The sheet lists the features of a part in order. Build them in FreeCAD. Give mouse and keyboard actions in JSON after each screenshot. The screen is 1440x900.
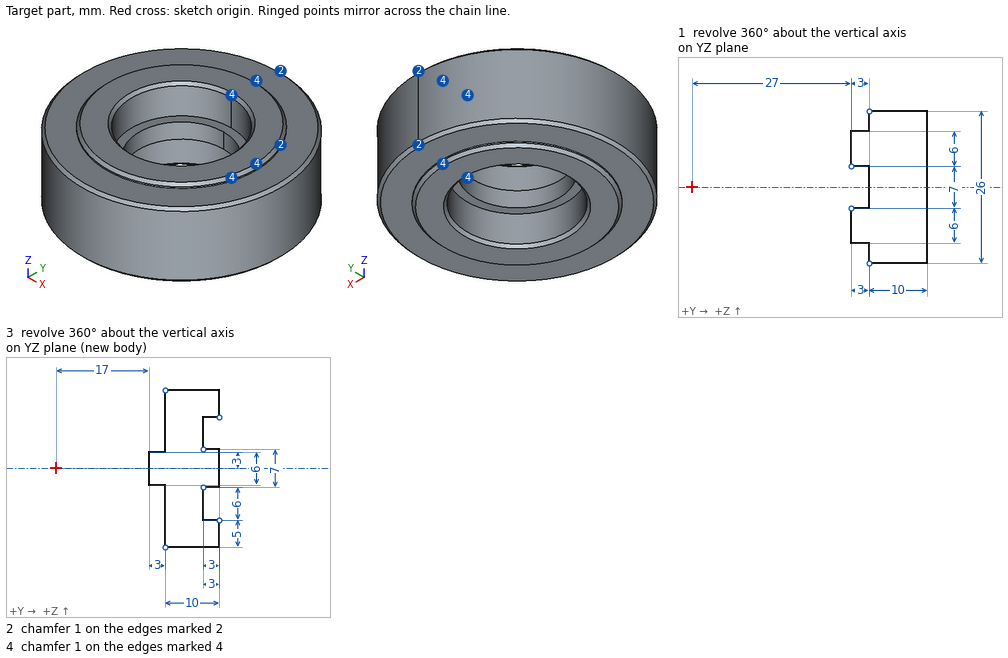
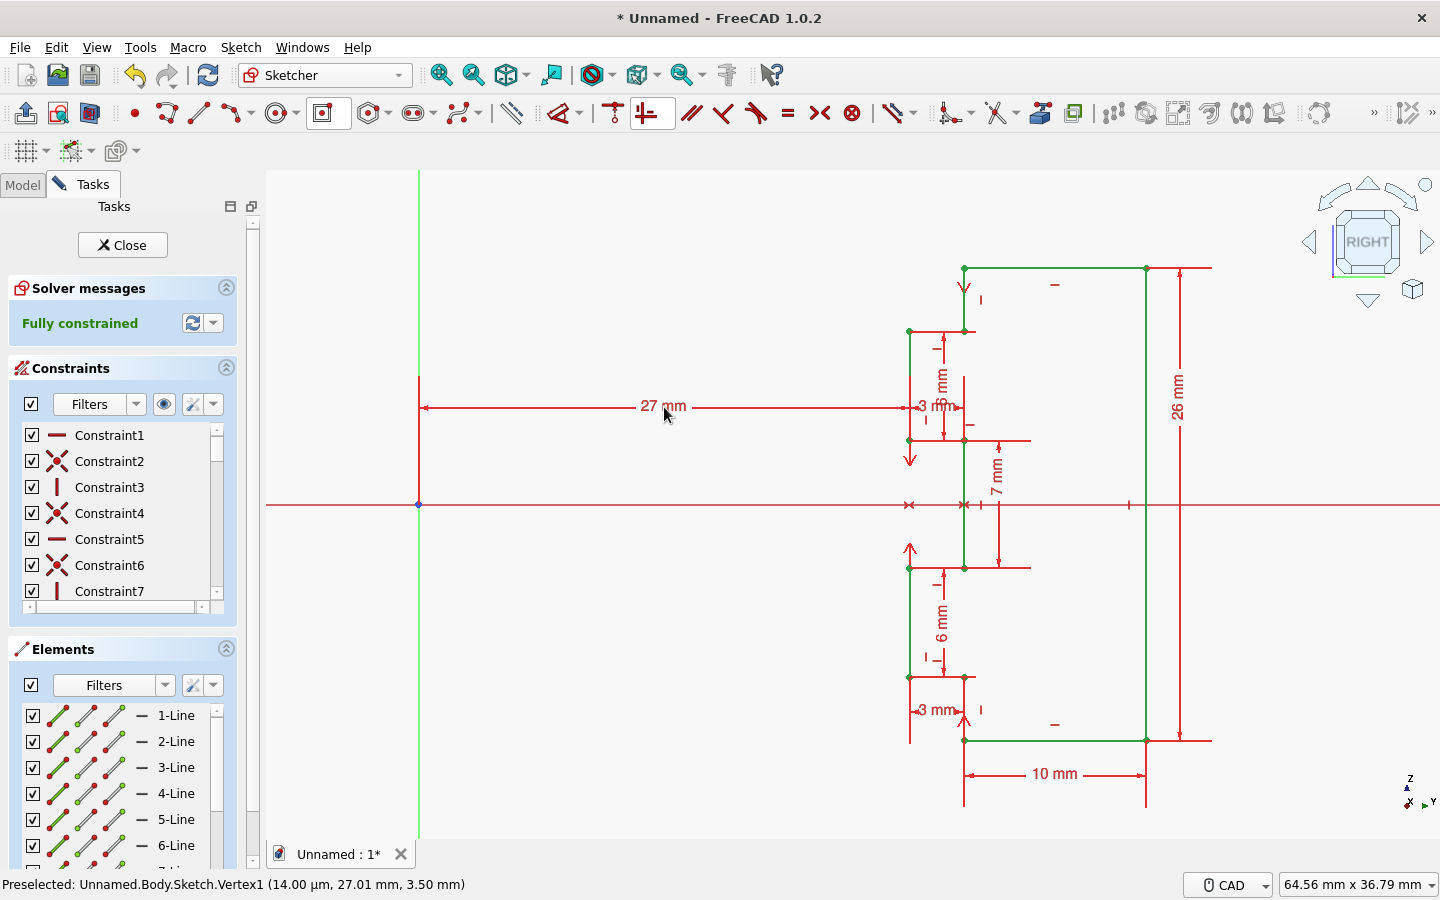
{"action": "left_click", "coordinate": [123, 245]}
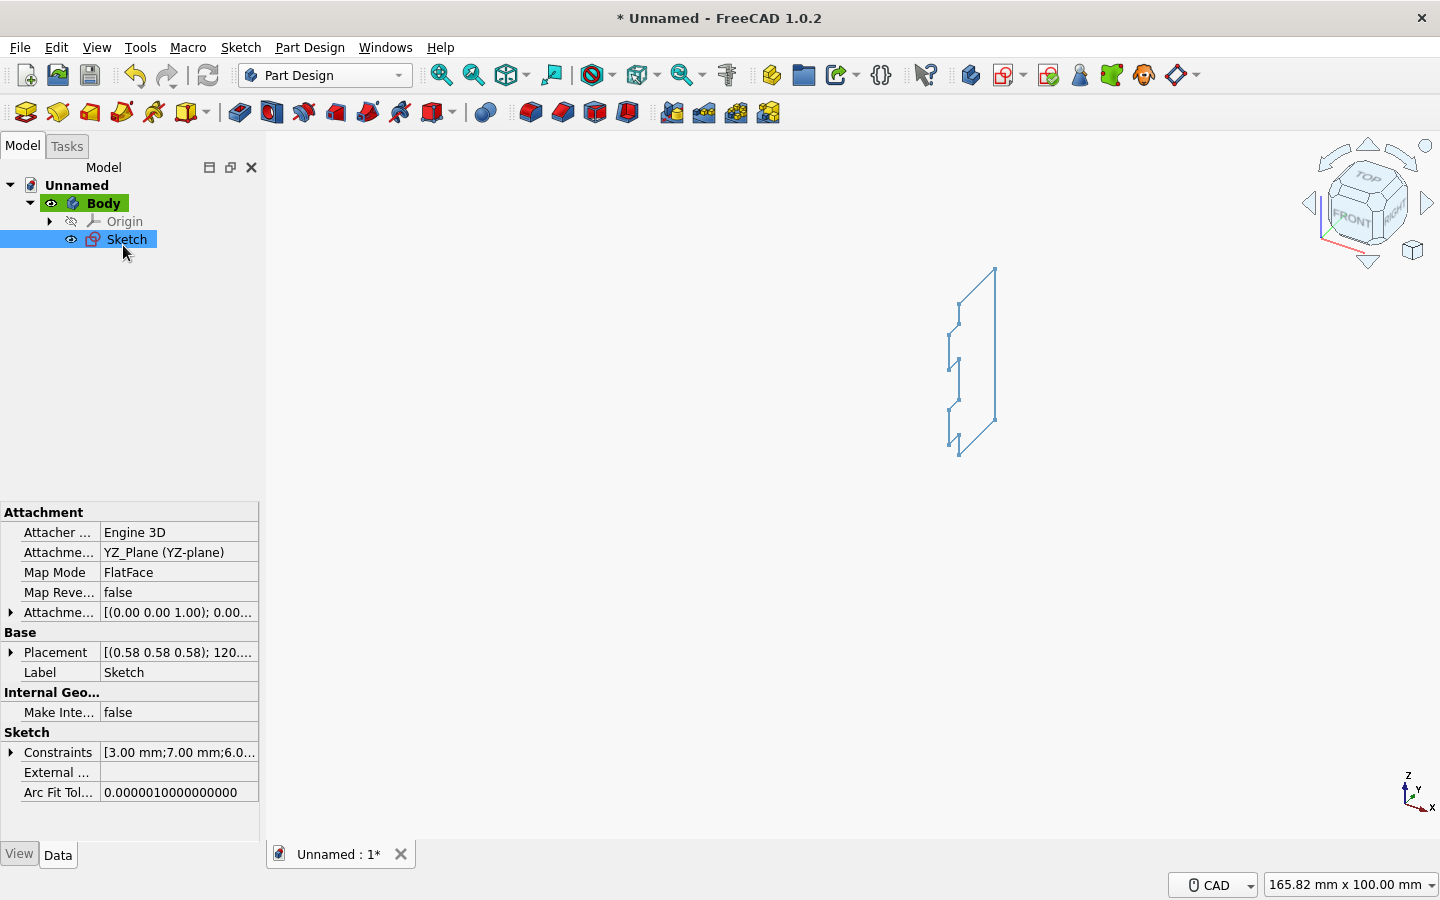
{"action": "left_click", "coordinate": [58, 112]}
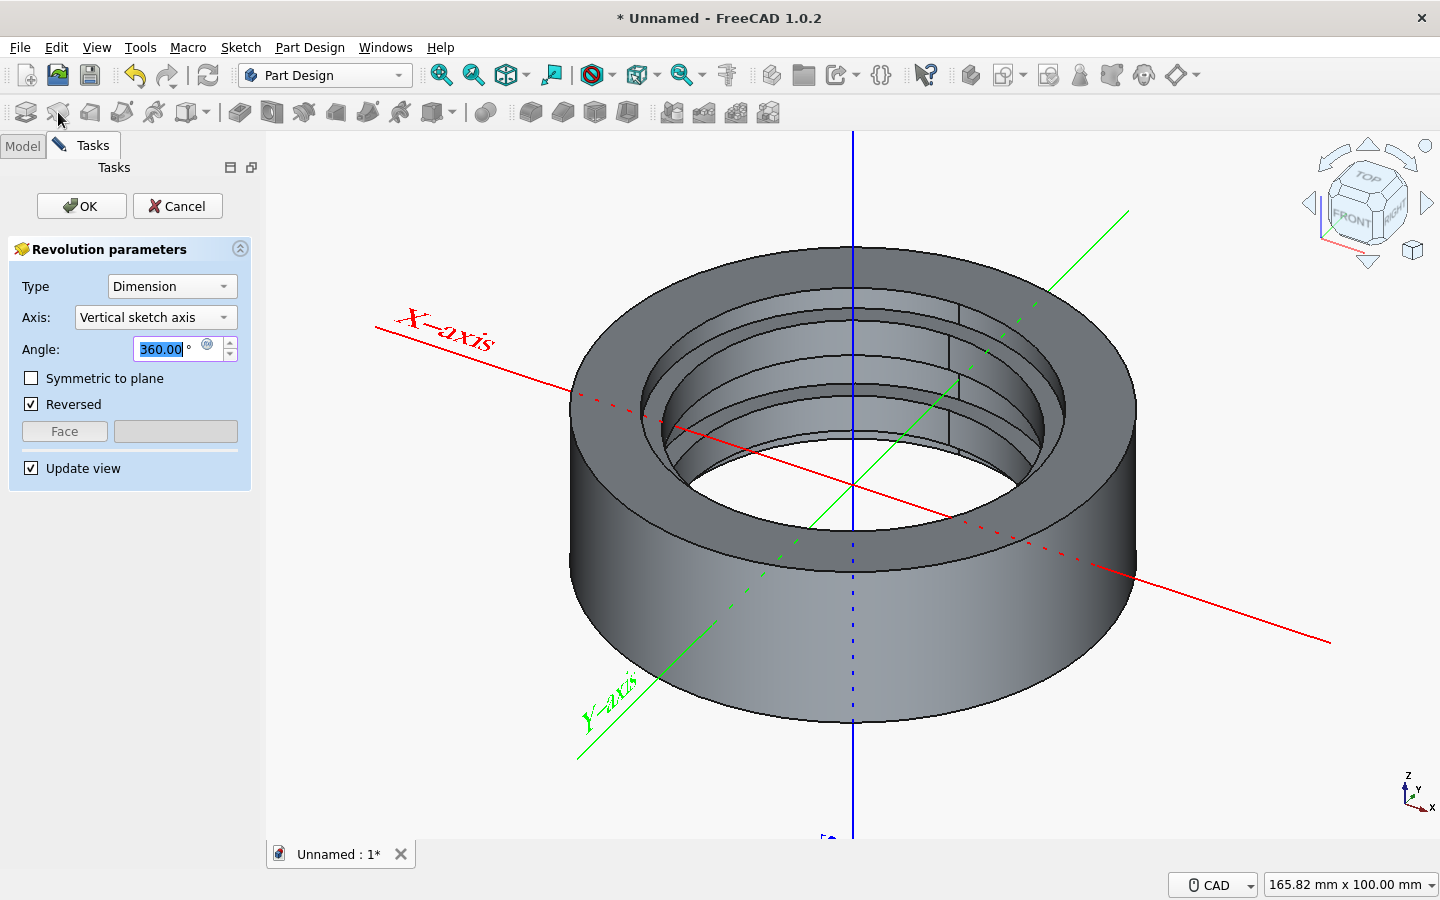
{"action": "left_click", "coordinate": [82, 206]}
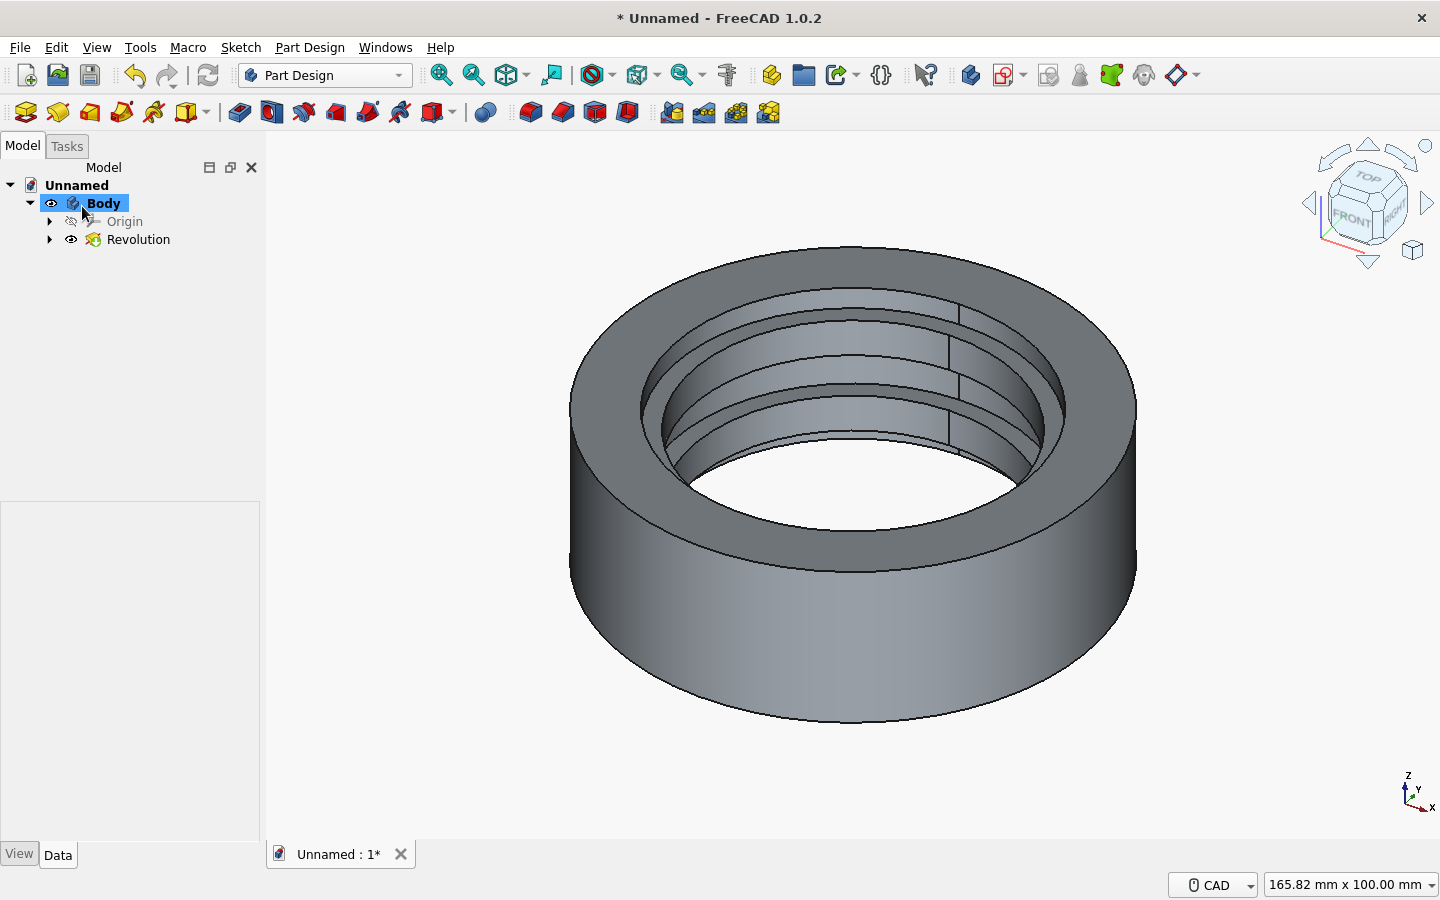
{"action": "left_click", "coordinate": [711, 549]}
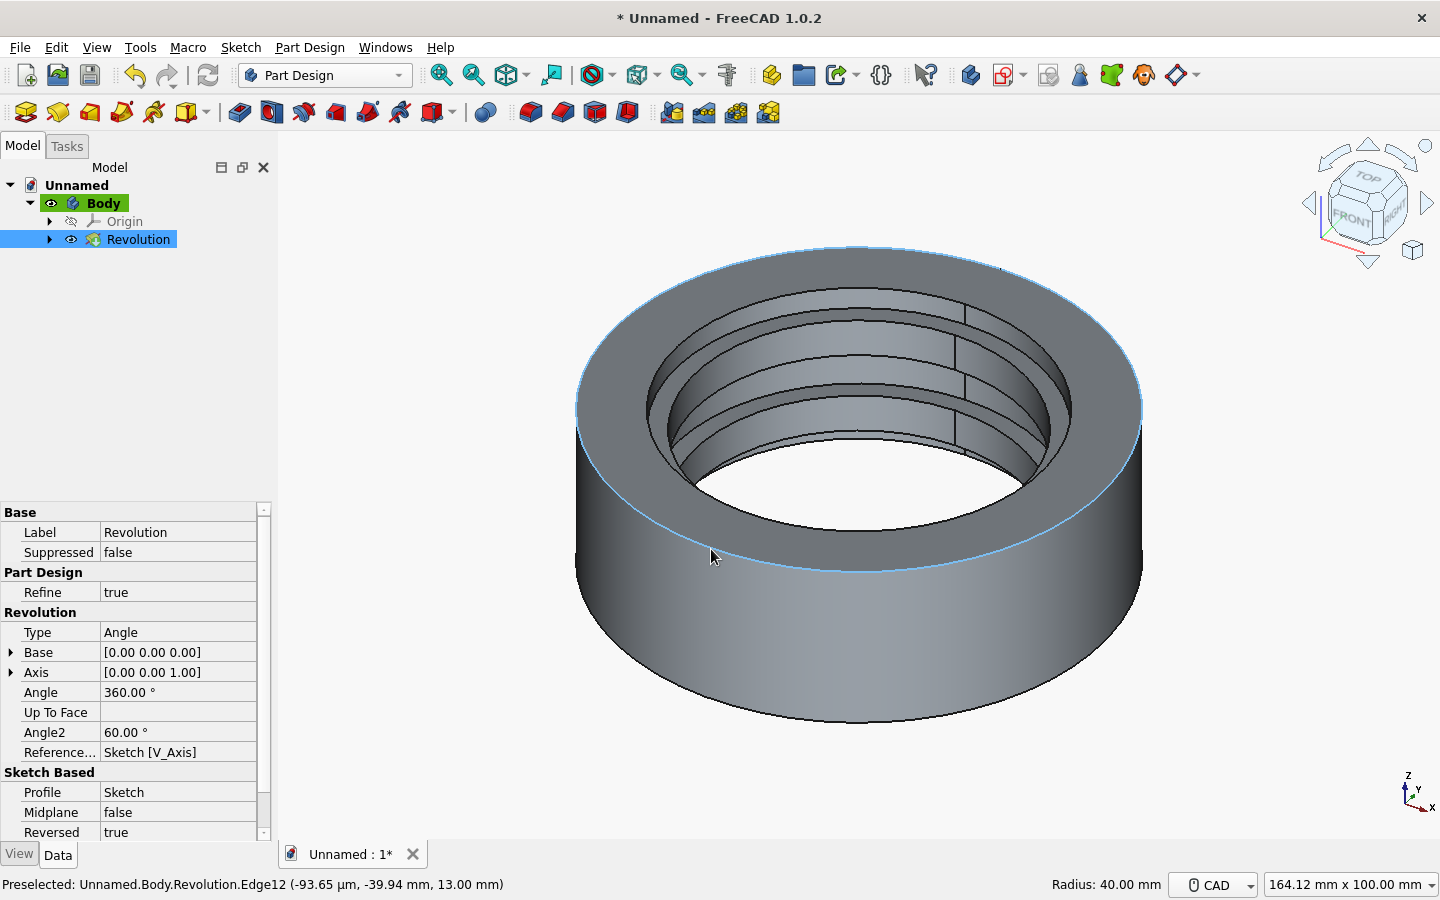
{"action": "key", "text": "0"}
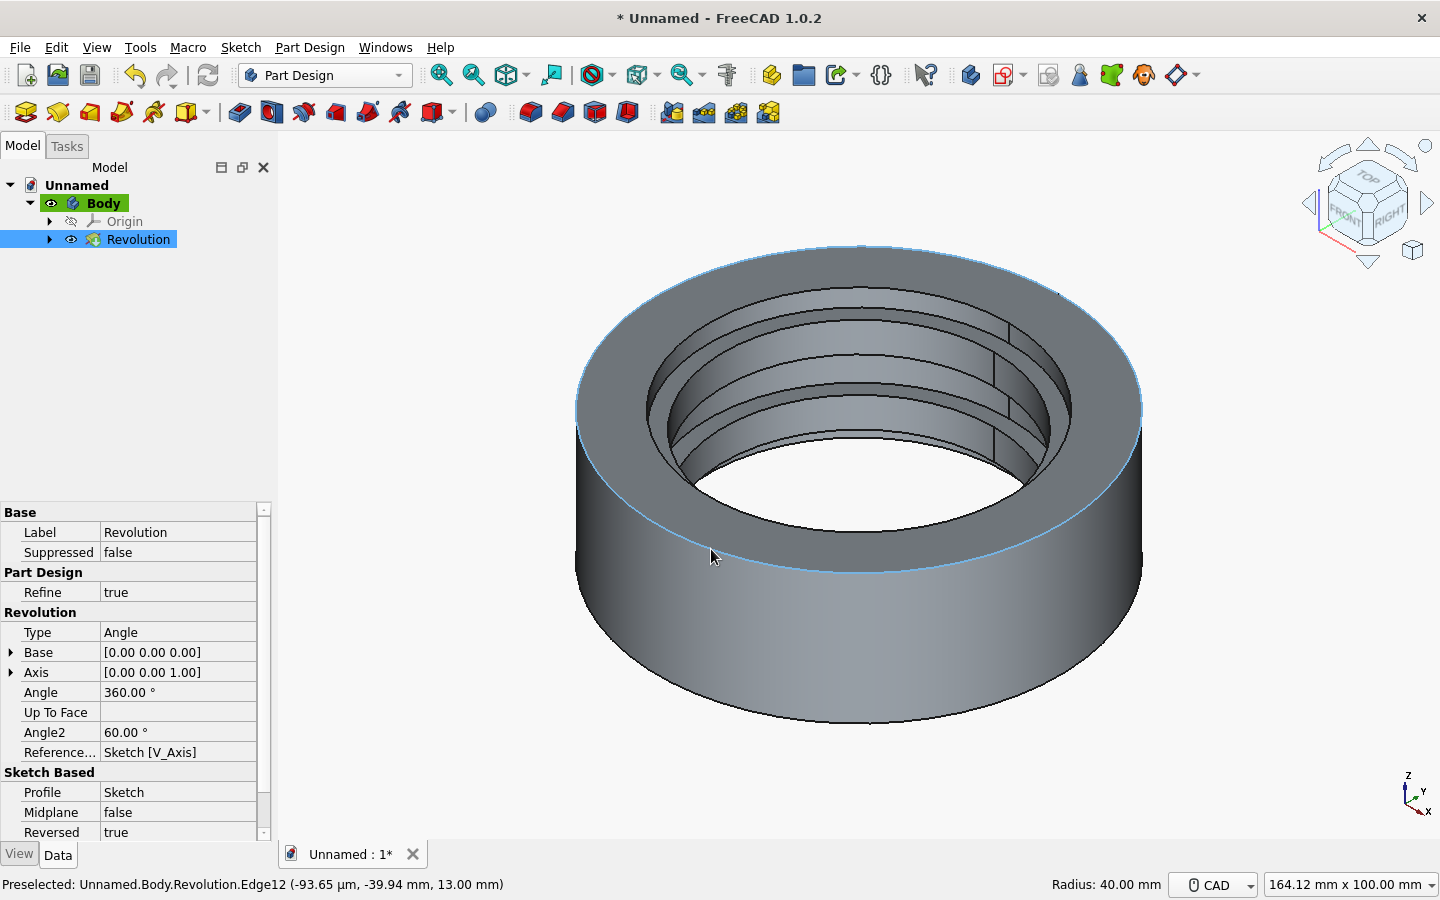
{"action": "key", "text": "2"}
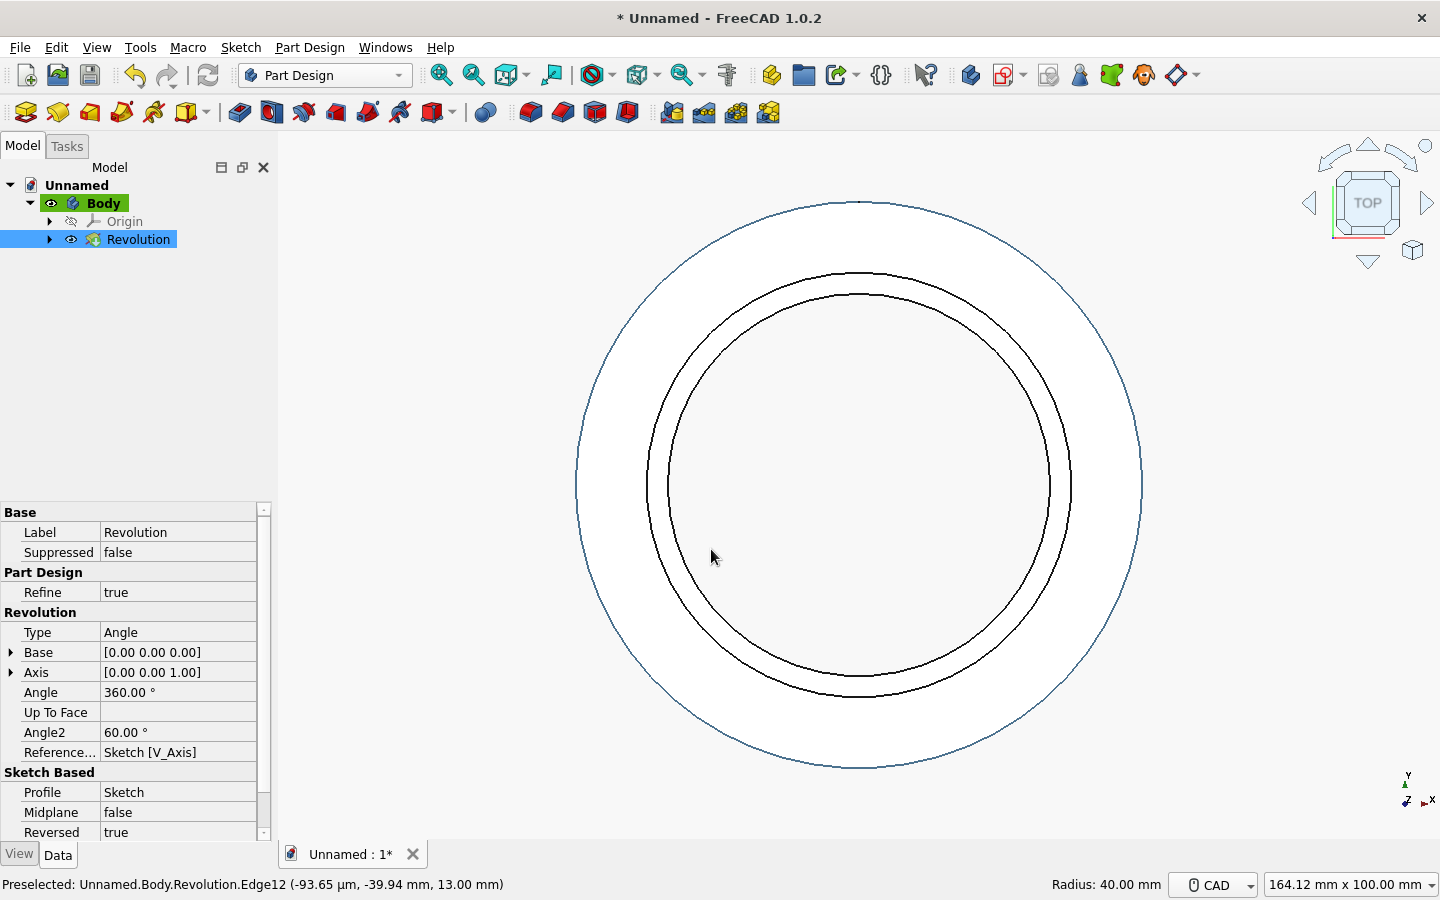
{"action": "key", "text": "1"}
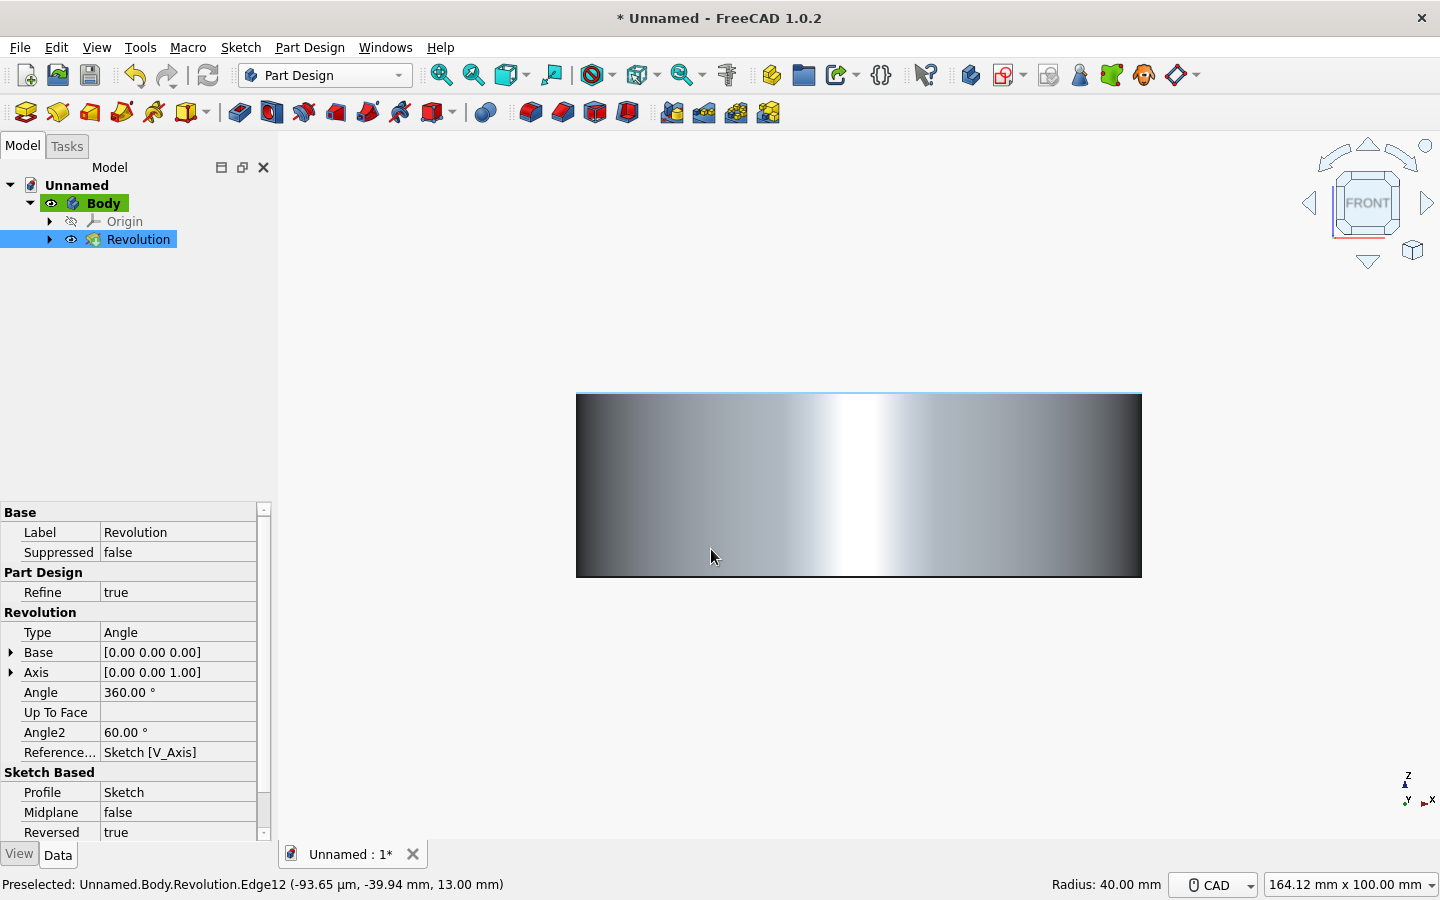
{"action": "left_click", "coordinate": [859, 576], "text": "ctrl"}